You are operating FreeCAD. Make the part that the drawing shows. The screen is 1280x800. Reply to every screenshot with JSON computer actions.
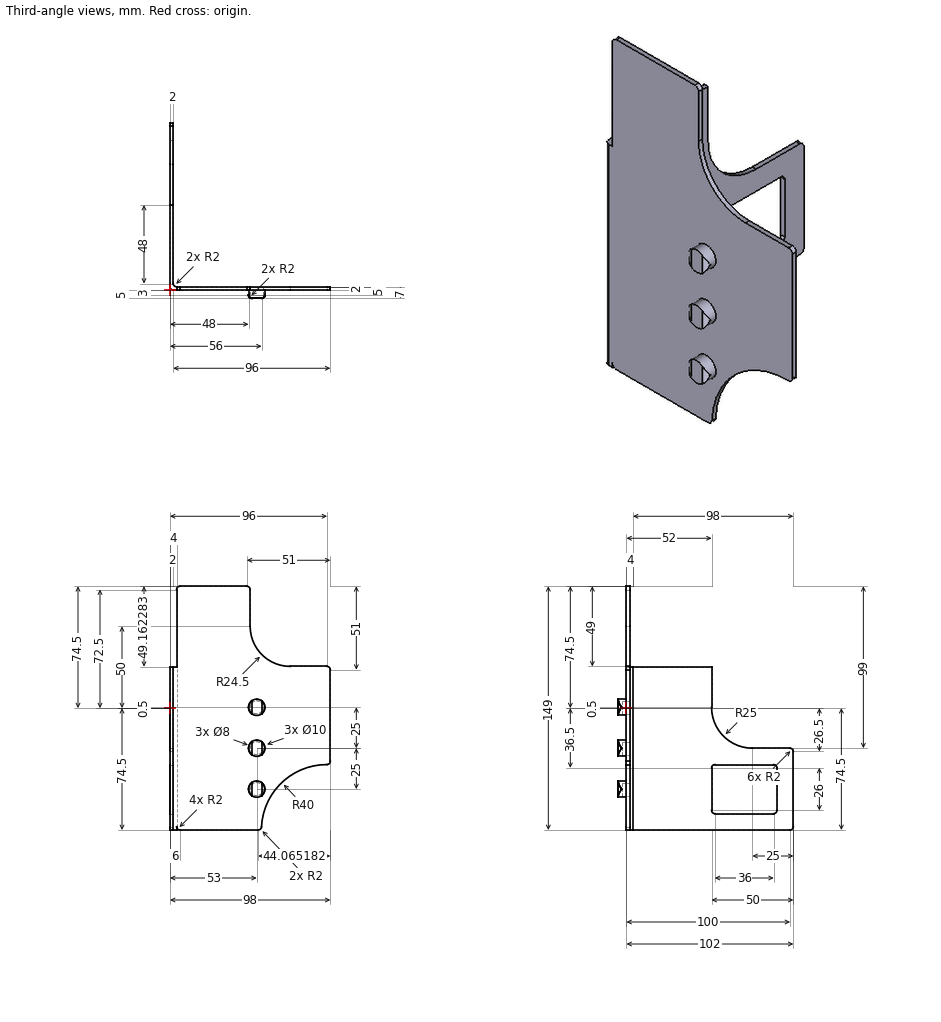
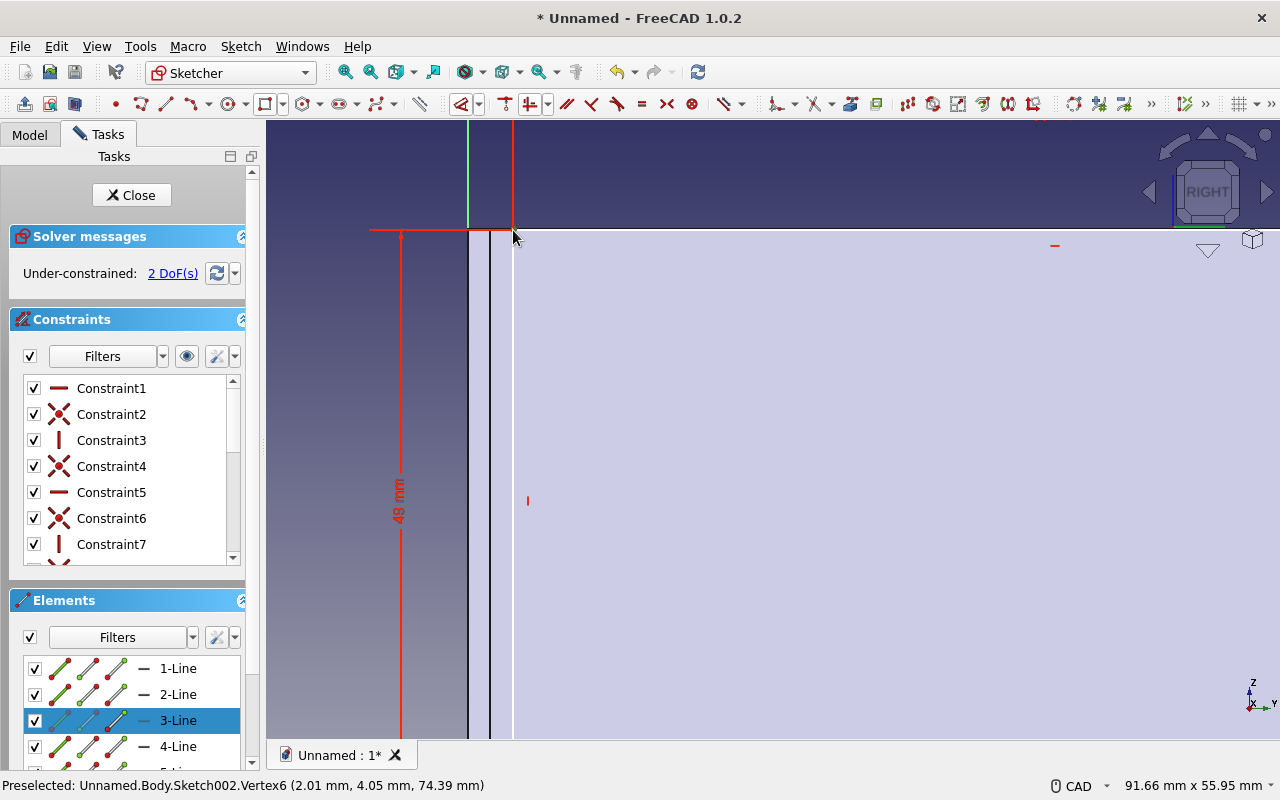
{"action": "key", "text": "l"}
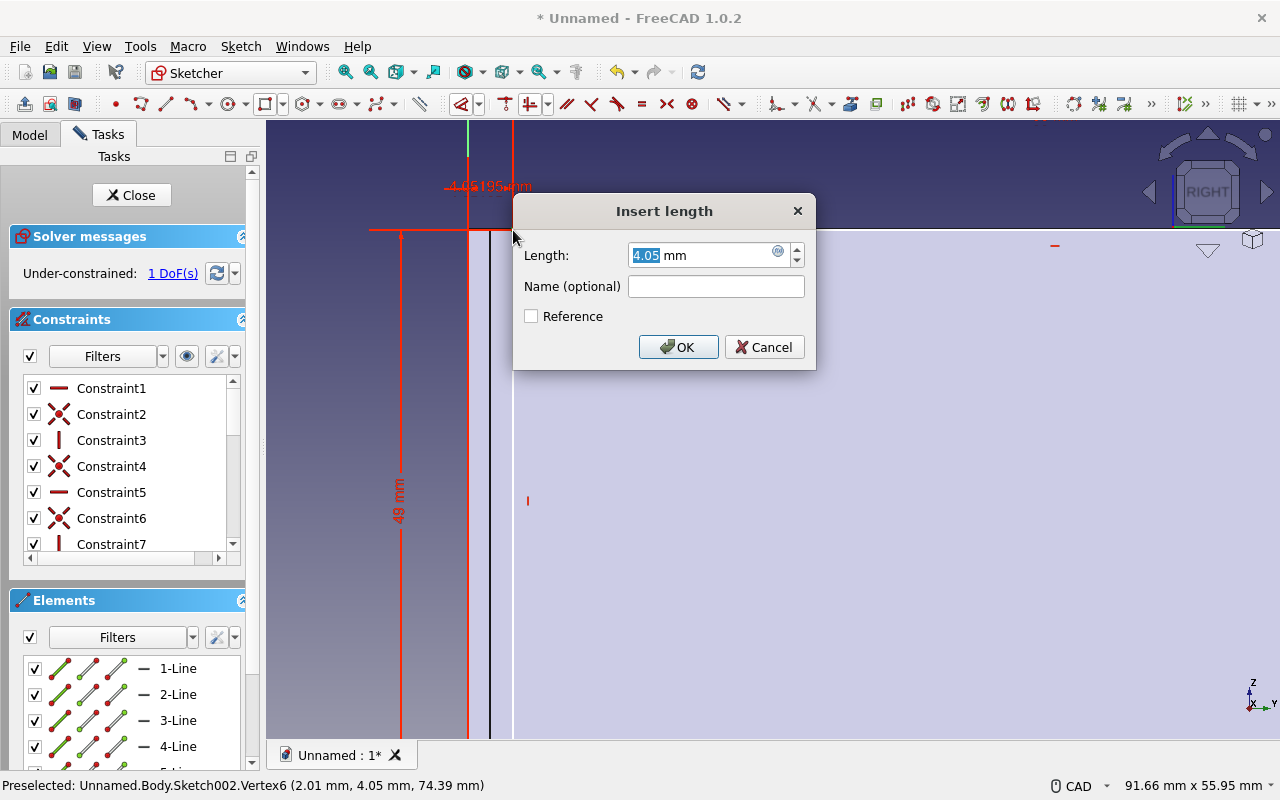
{"action": "type", "text": "4"}
{"action": "key", "text": "Return"}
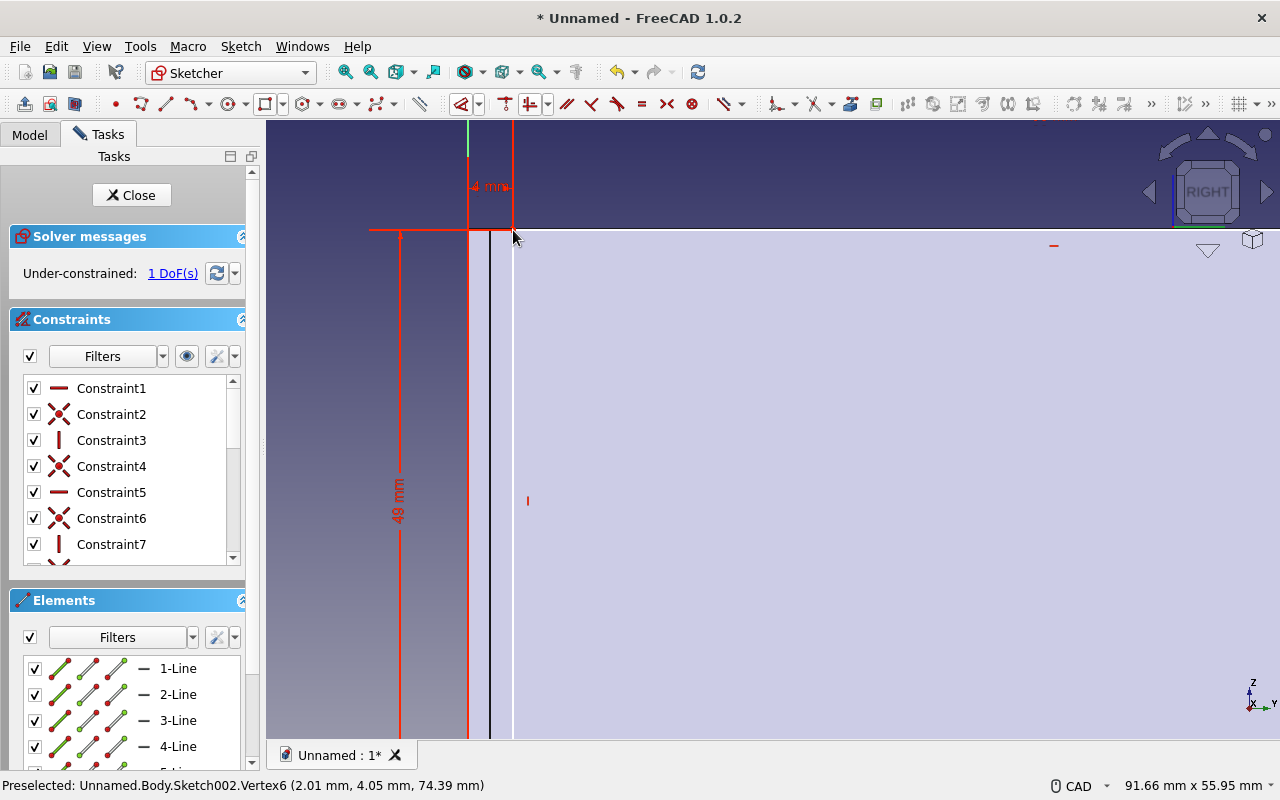
{"action": "scroll", "coordinate": [514, 228], "scroll_direction": "down", "scroll_amount": 5}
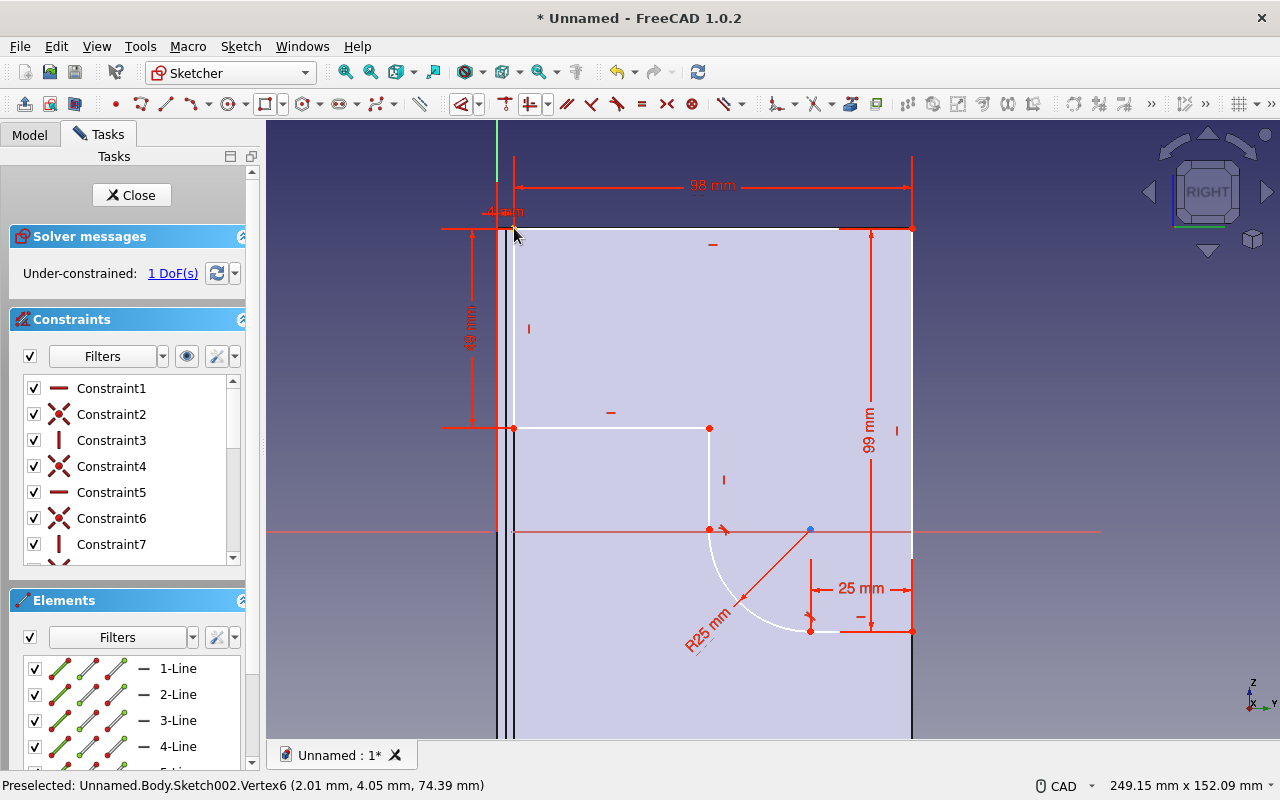
{"action": "scroll", "coordinate": [709, 530], "scroll_direction": "up", "scroll_amount": 15}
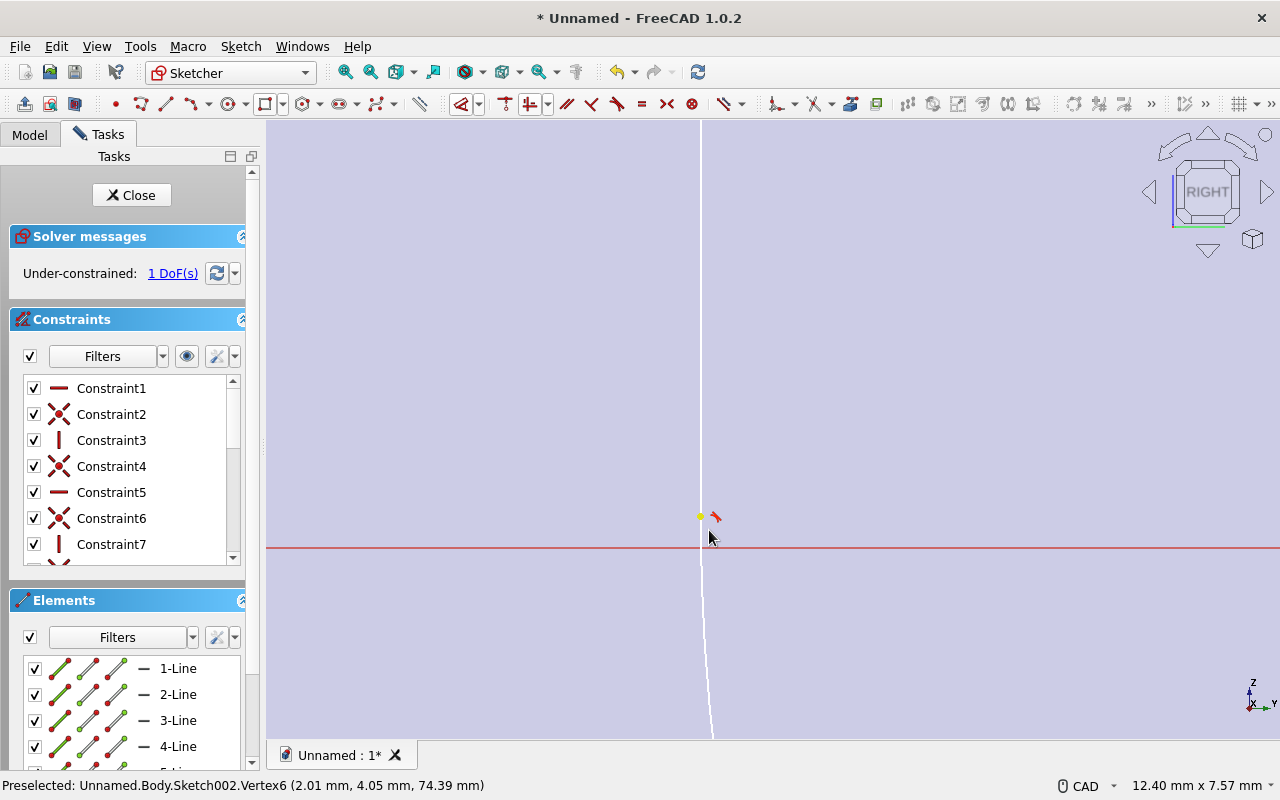
{"action": "left_click", "coordinate": [701, 516]}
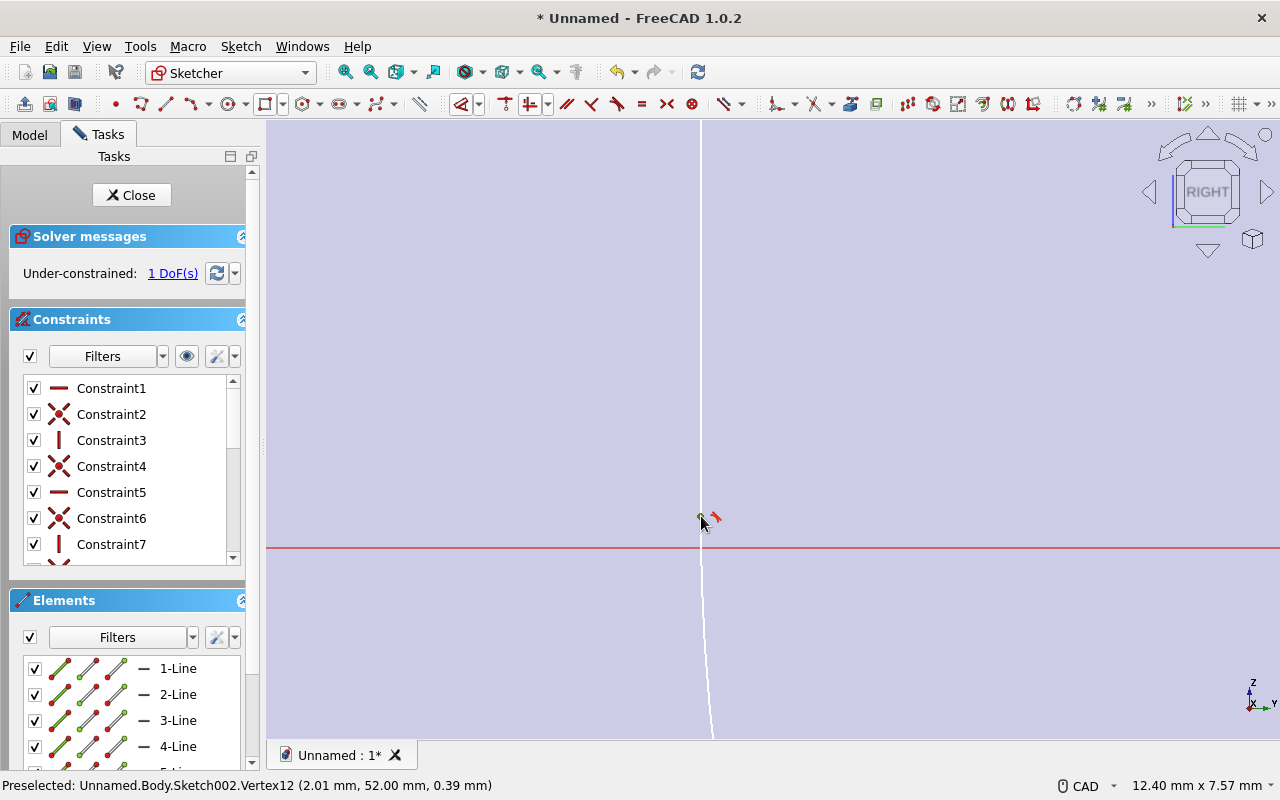
{"action": "key", "text": "i"}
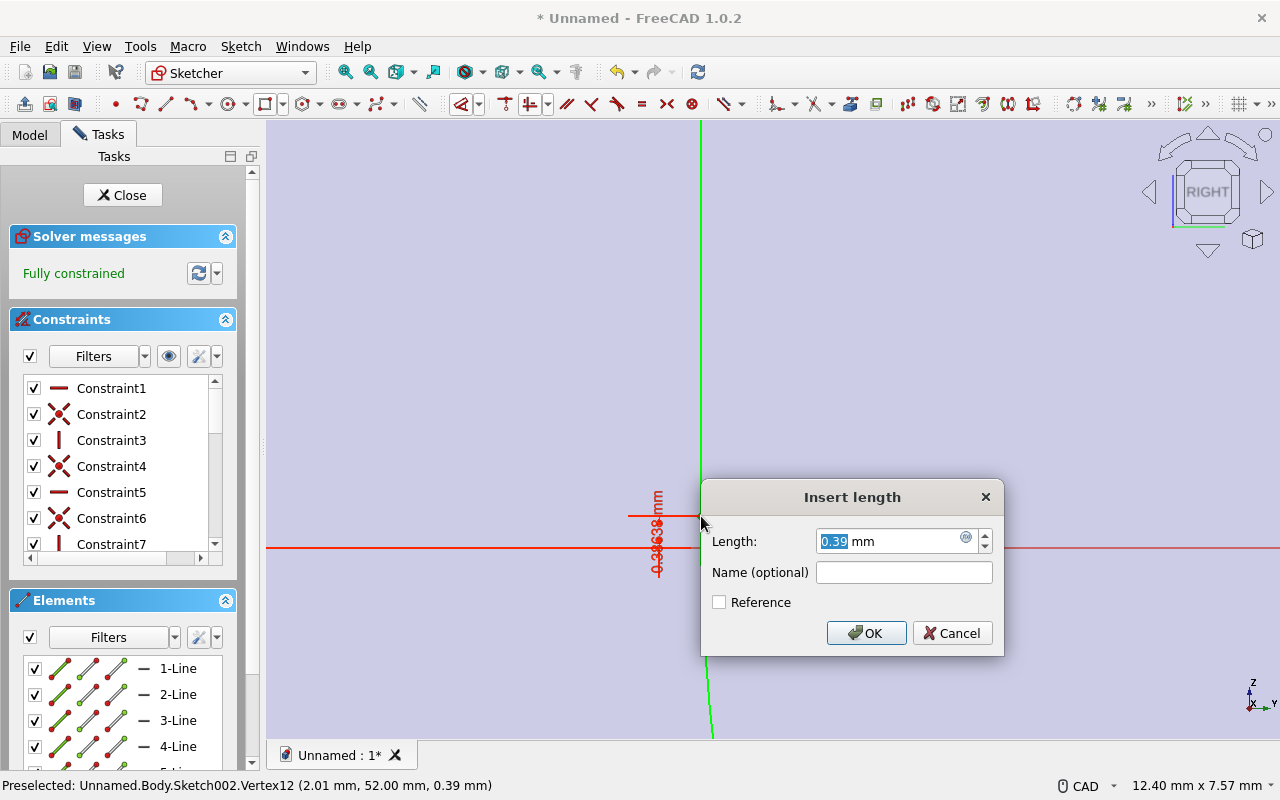
{"action": "type", "text": "0.5"}
{"action": "key", "text": "Return"}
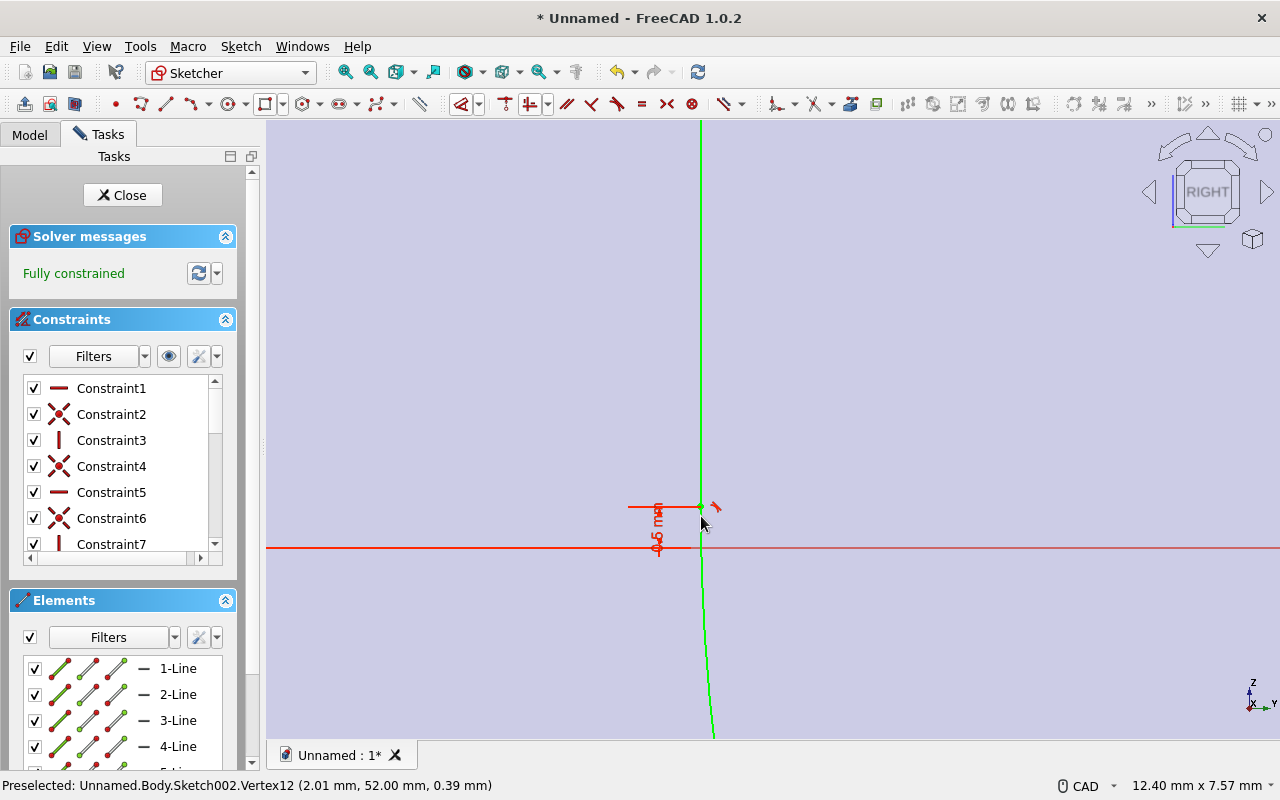
{"action": "left_click", "coordinate": [123, 195]}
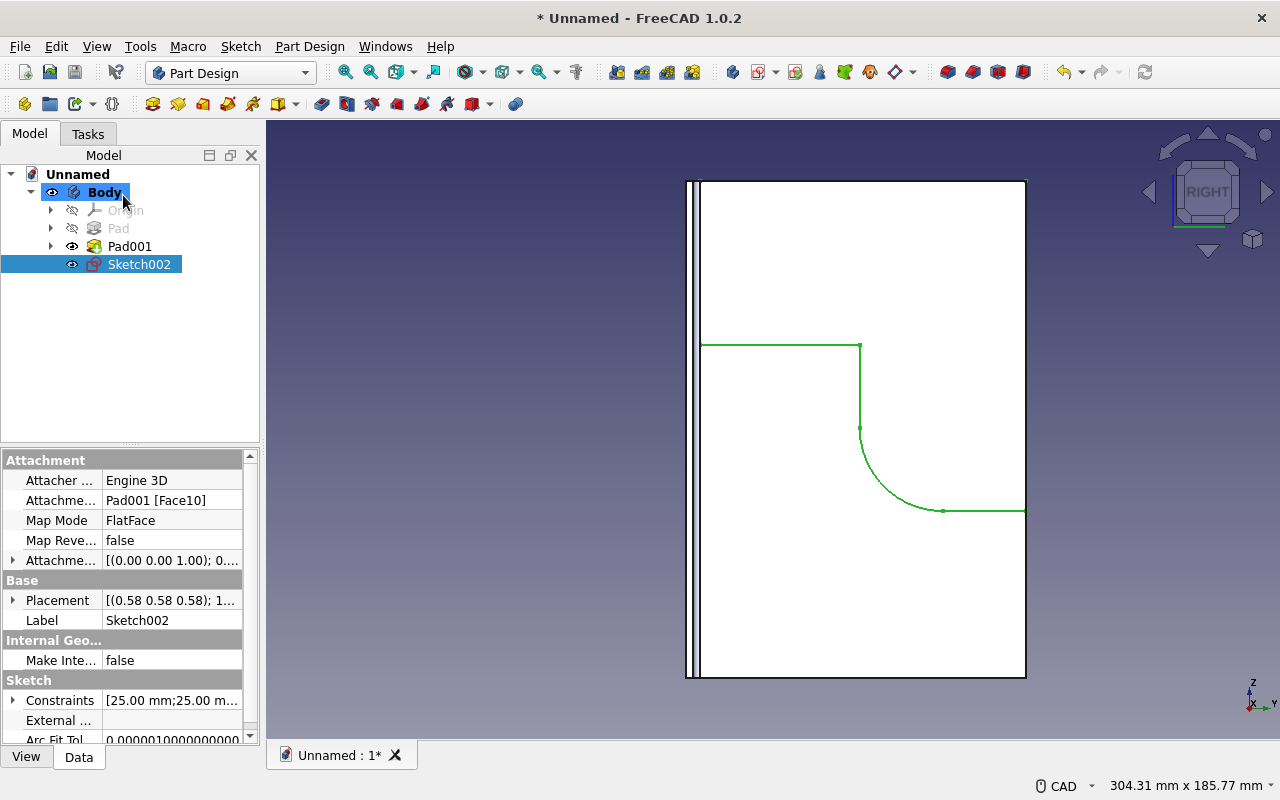
{"action": "left_click", "coordinate": [322, 104]}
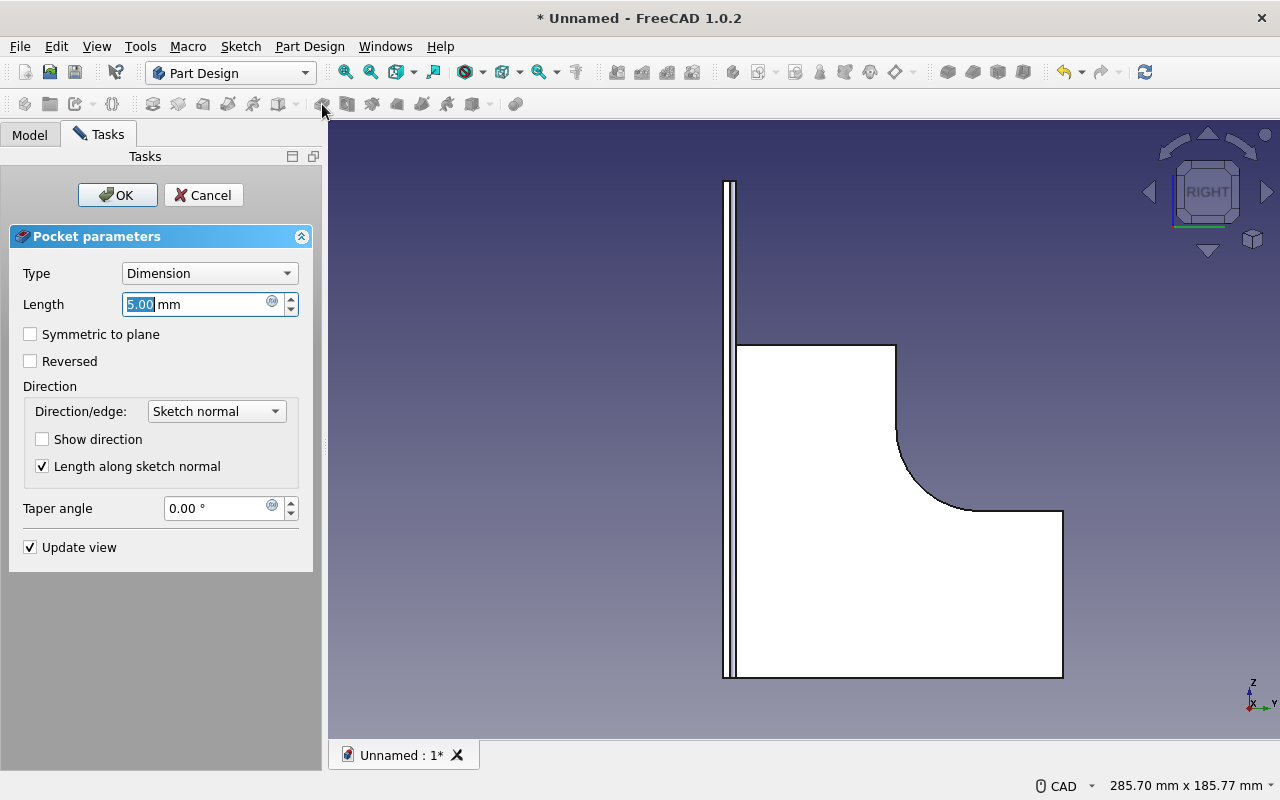
{"action": "type", "text": "2"}
{"action": "key", "text": "Tab"}